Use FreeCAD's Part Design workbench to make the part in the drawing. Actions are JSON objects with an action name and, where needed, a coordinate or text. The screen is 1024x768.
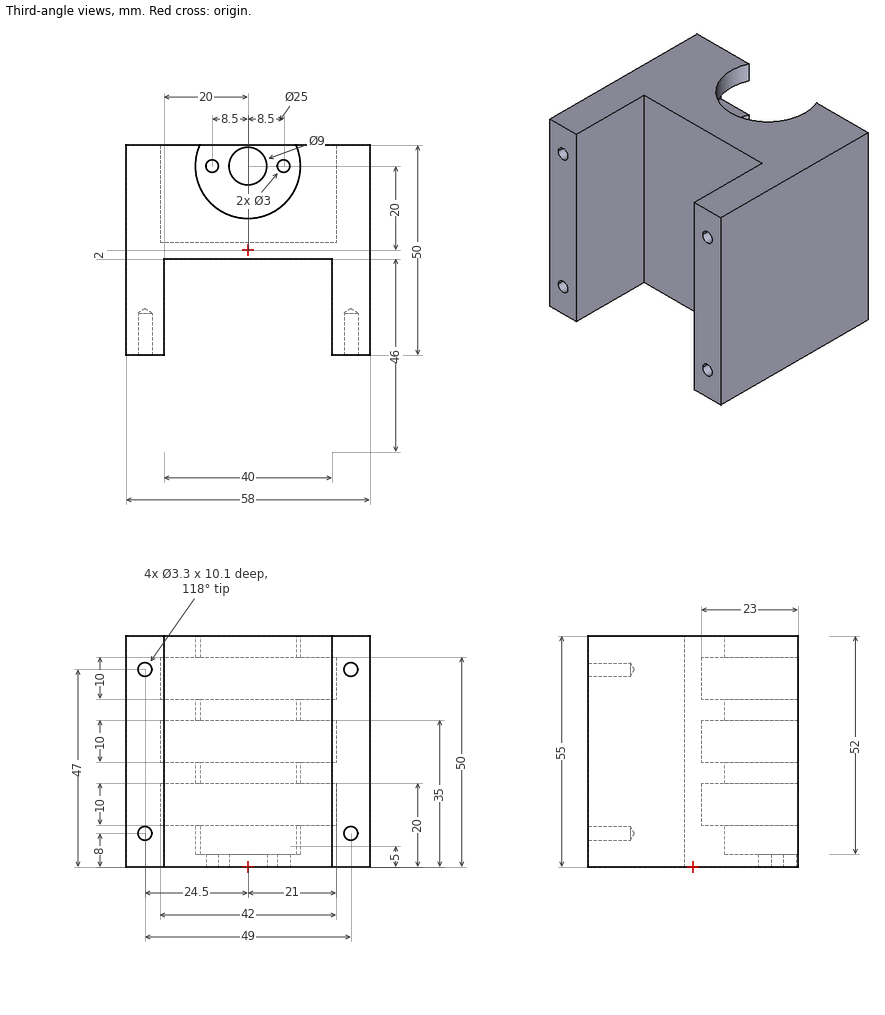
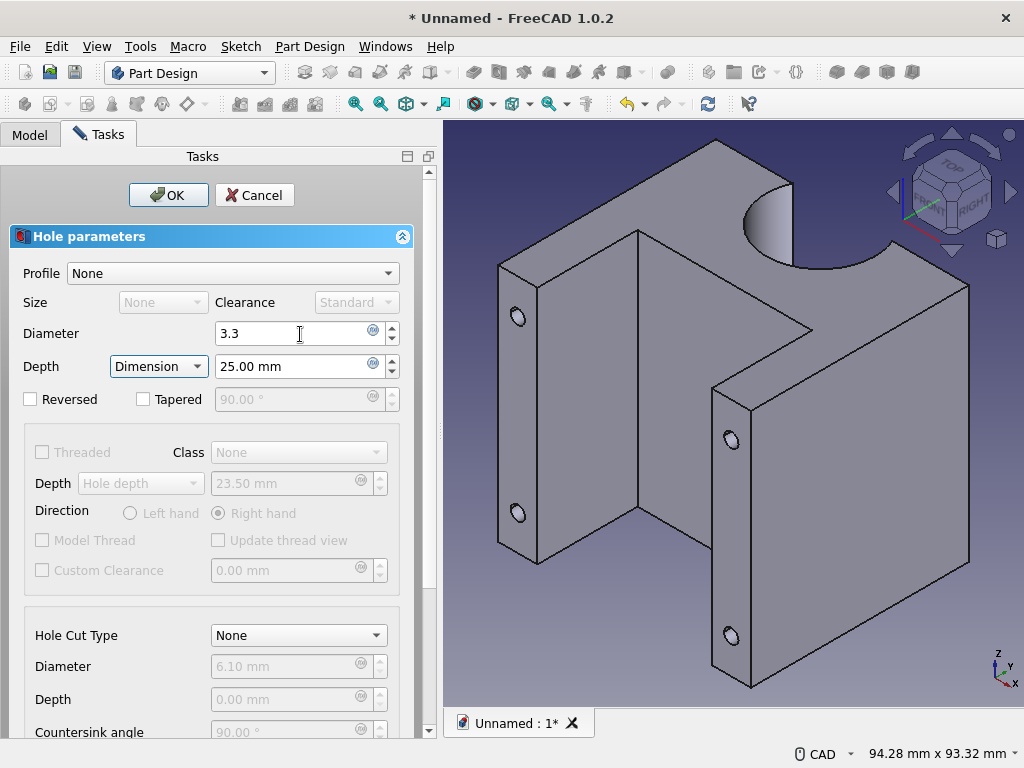
{"action": "triple_click", "coordinate": [300, 366]}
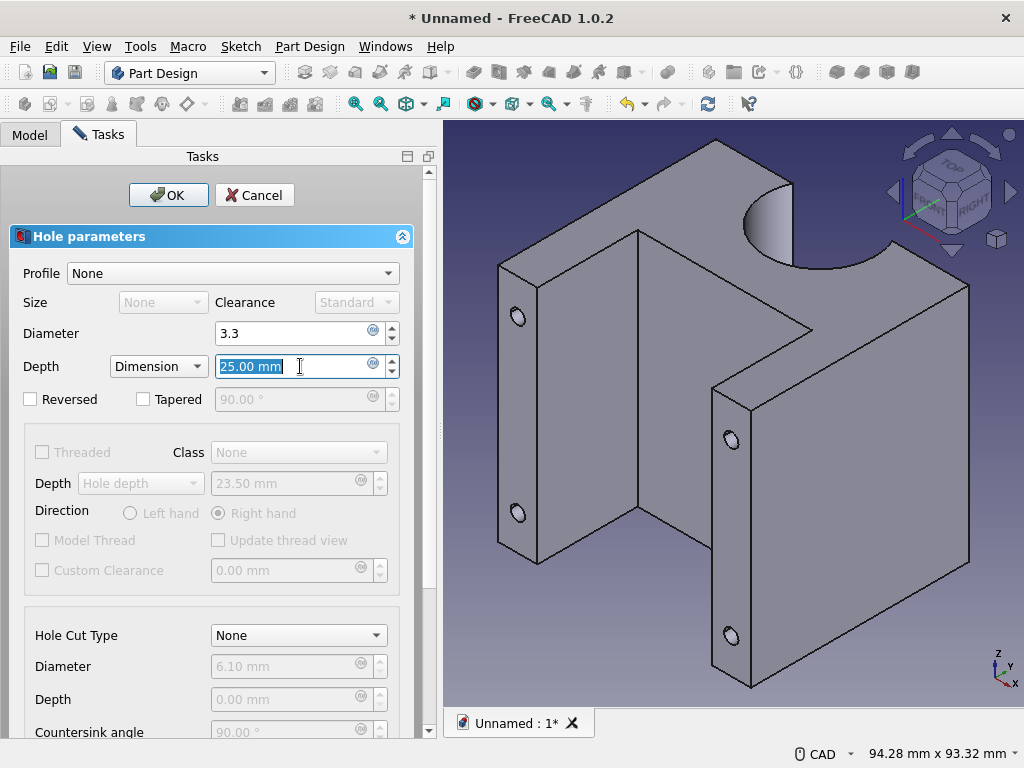
{"action": "type", "text": "10.1"}
{"action": "key", "text": "Tab"}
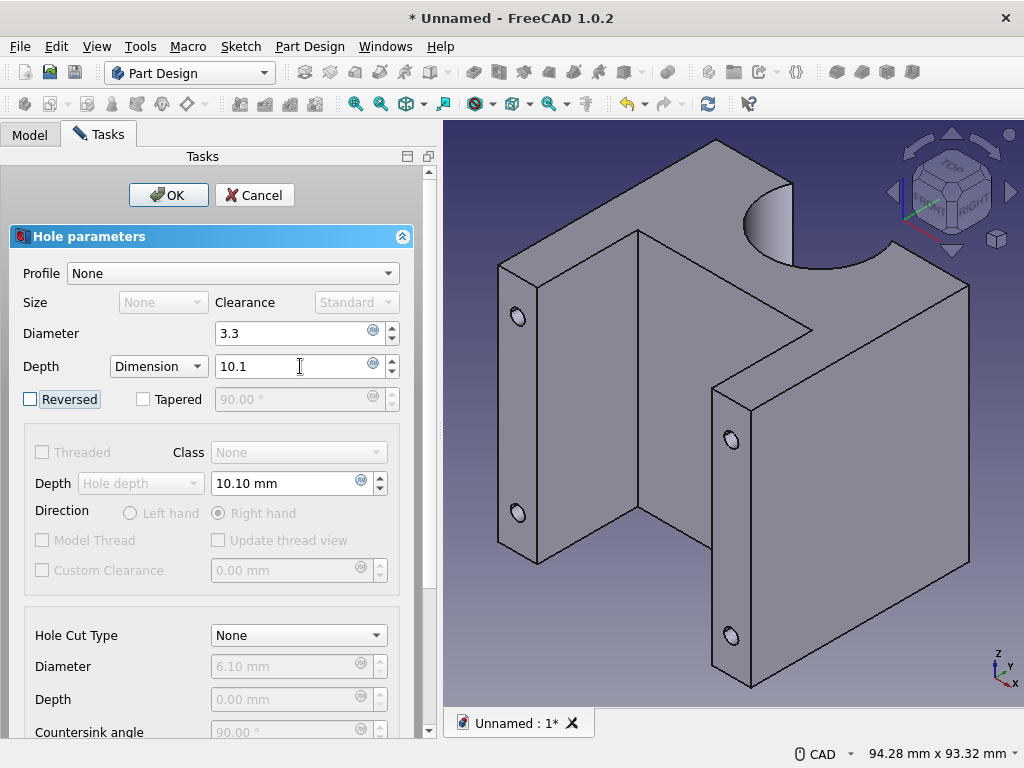
{"action": "left_click", "coordinate": [169, 195]}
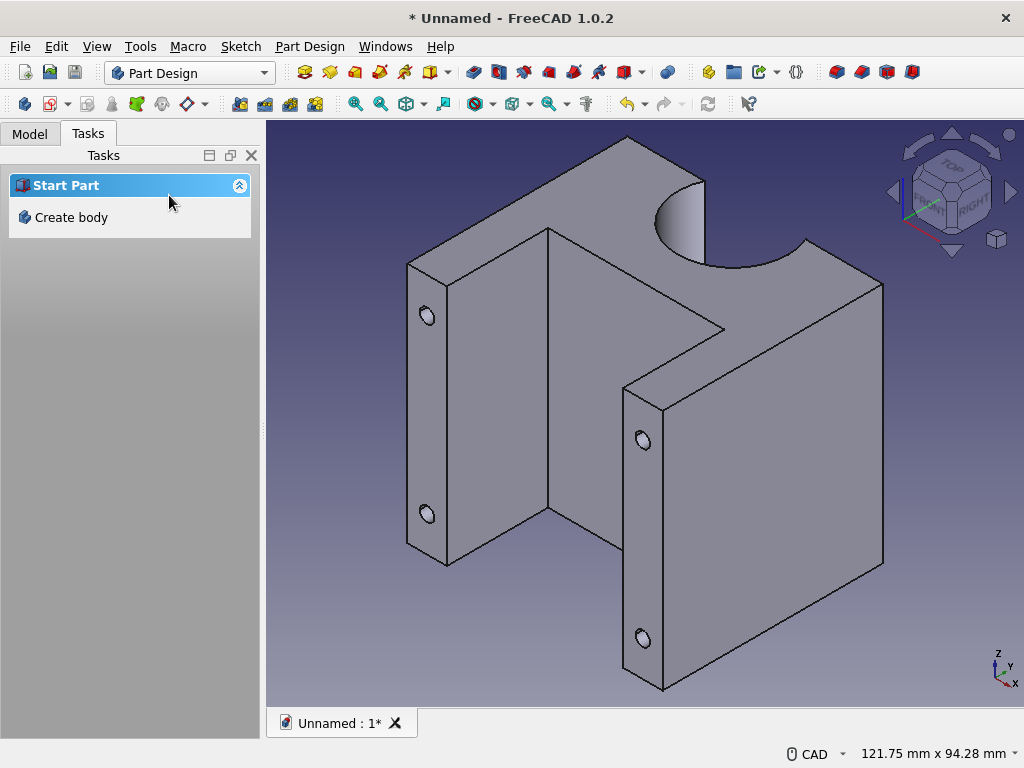
{"action": "key", "text": "4"}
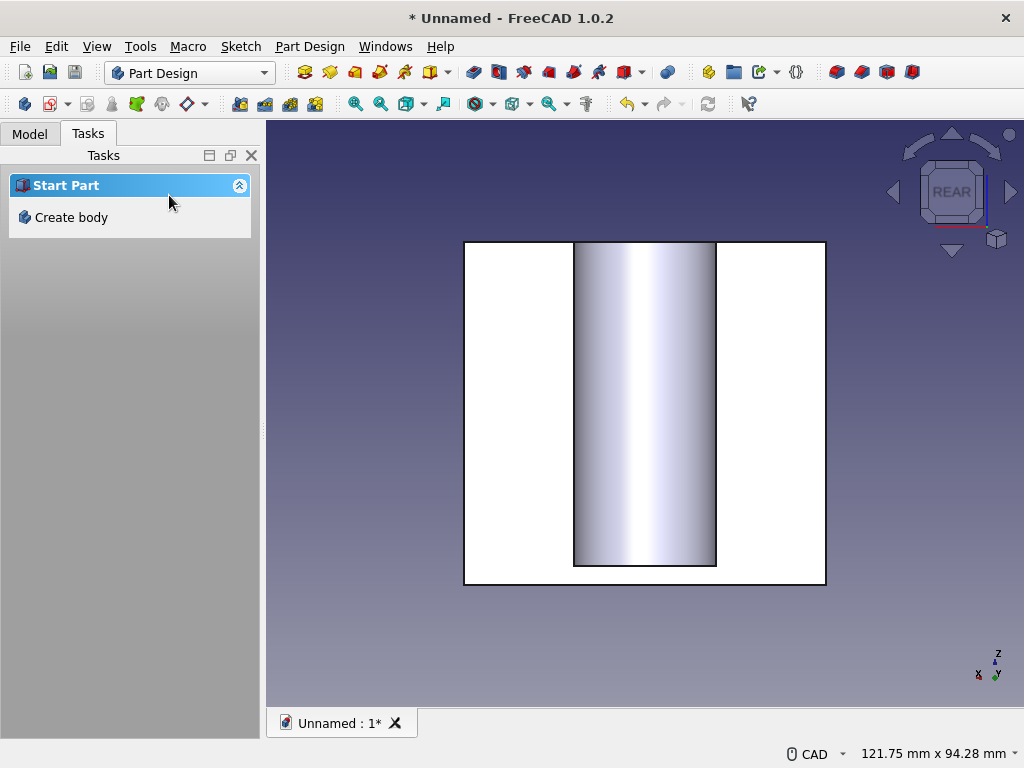
{"action": "left_click", "coordinate": [542, 315]}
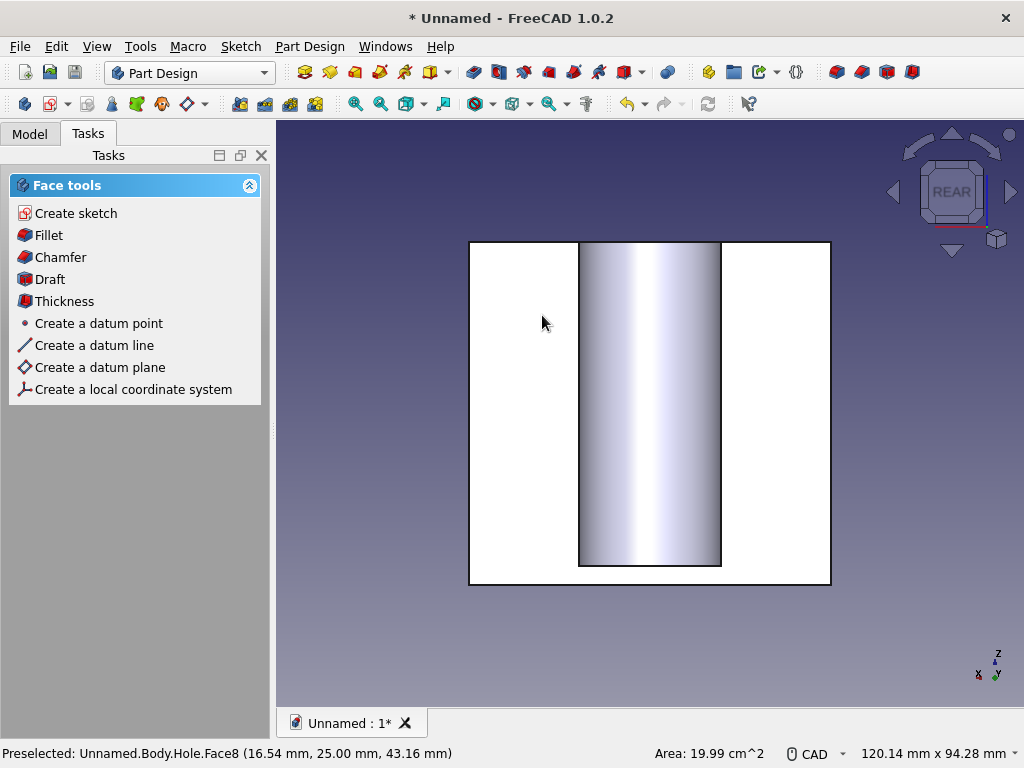
{"action": "left_click", "coordinate": [50, 104]}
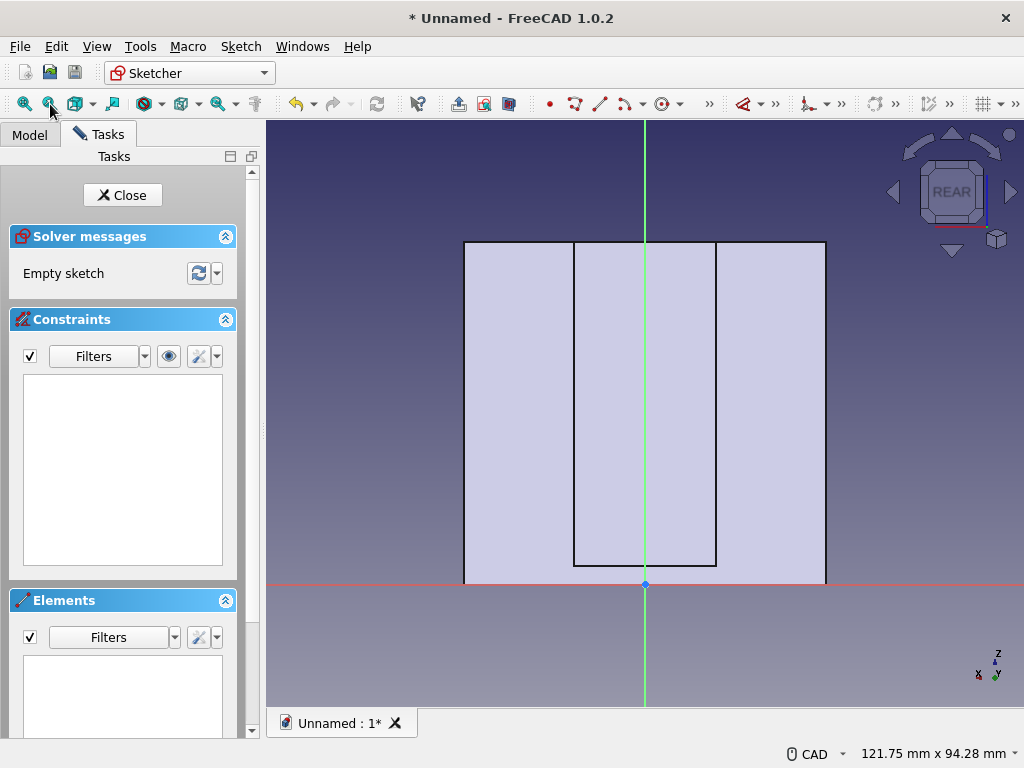
{"action": "key", "text": "g r"}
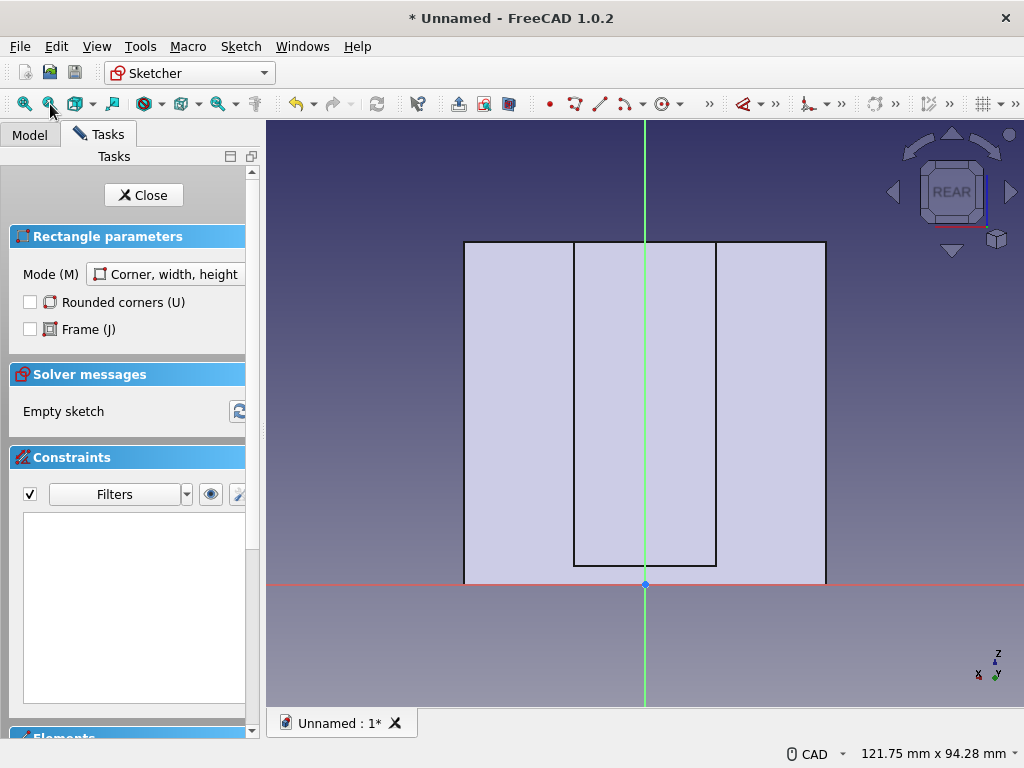
{"action": "left_click", "coordinate": [514, 460]}
{"action": "mouse_move", "coordinate": [776, 522]}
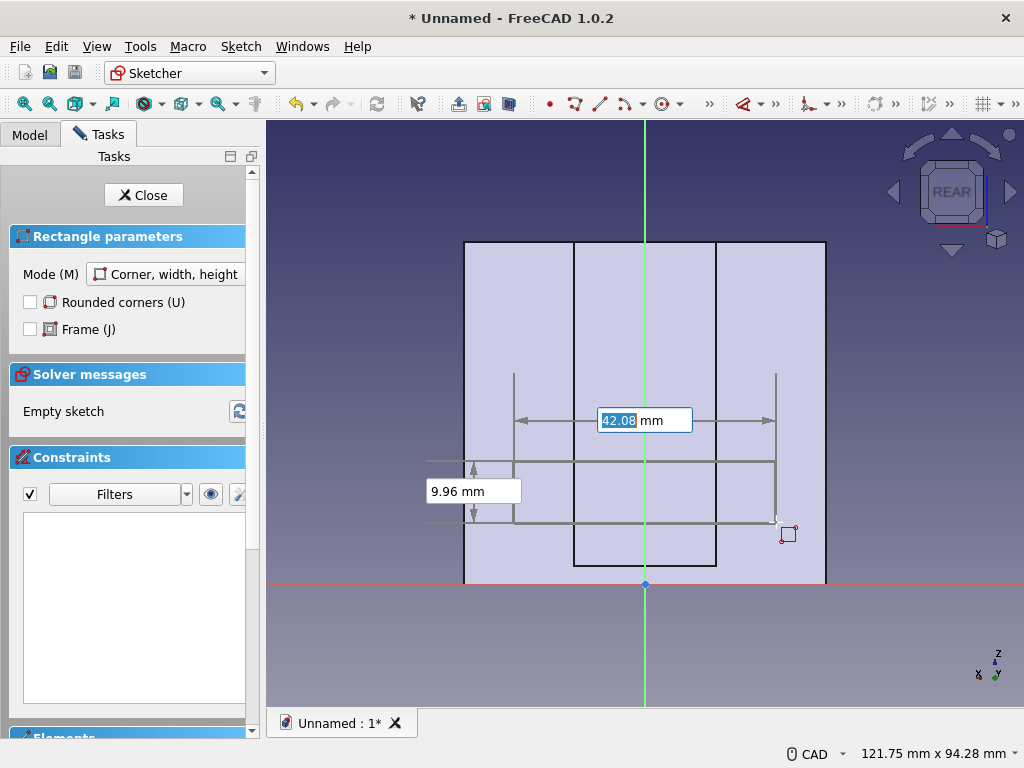
{"action": "type", "text": "42"}
{"action": "key", "text": "Tab"}
{"action": "type", "text": "10"}
{"action": "key", "text": "Return"}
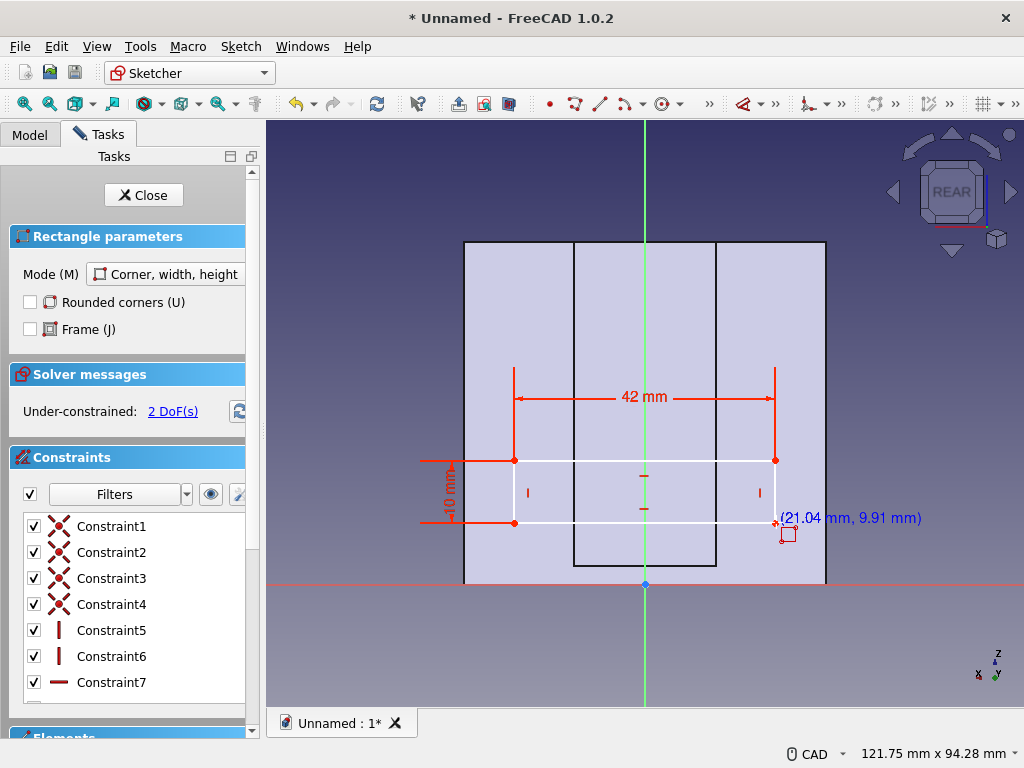
{"action": "left_click", "coordinate": [514, 367]}
{"action": "mouse_move", "coordinate": [776, 429]}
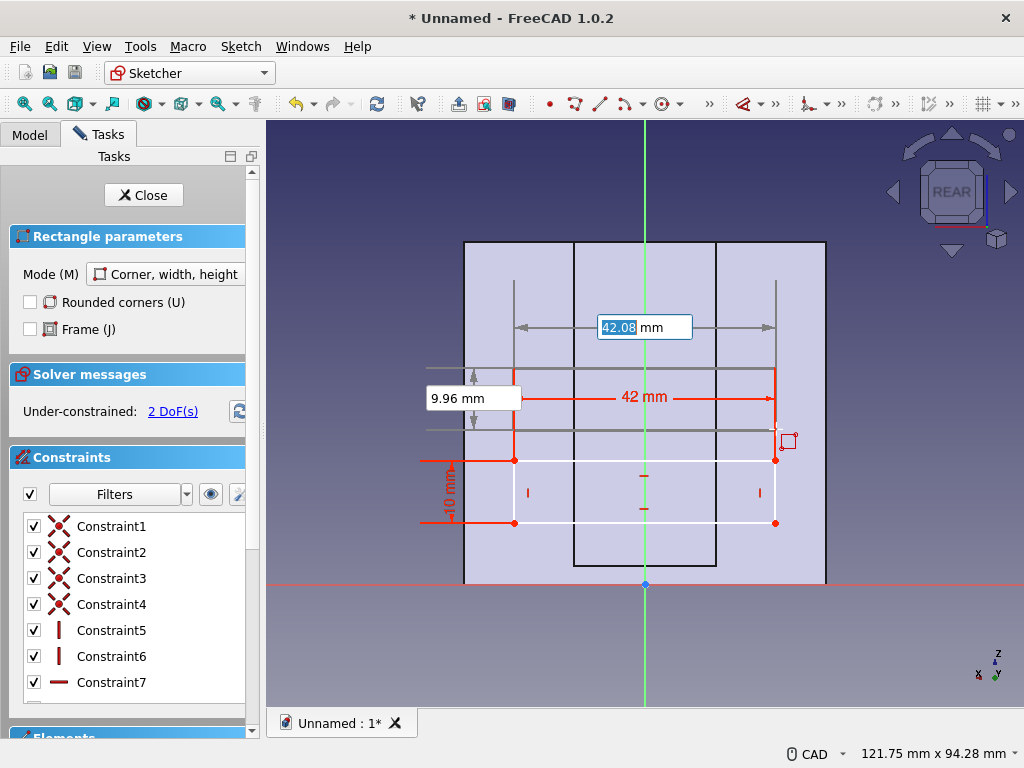
{"action": "type", "text": "42"}
{"action": "key", "text": "Tab"}
{"action": "type", "text": "10"}
{"action": "key", "text": "Return"}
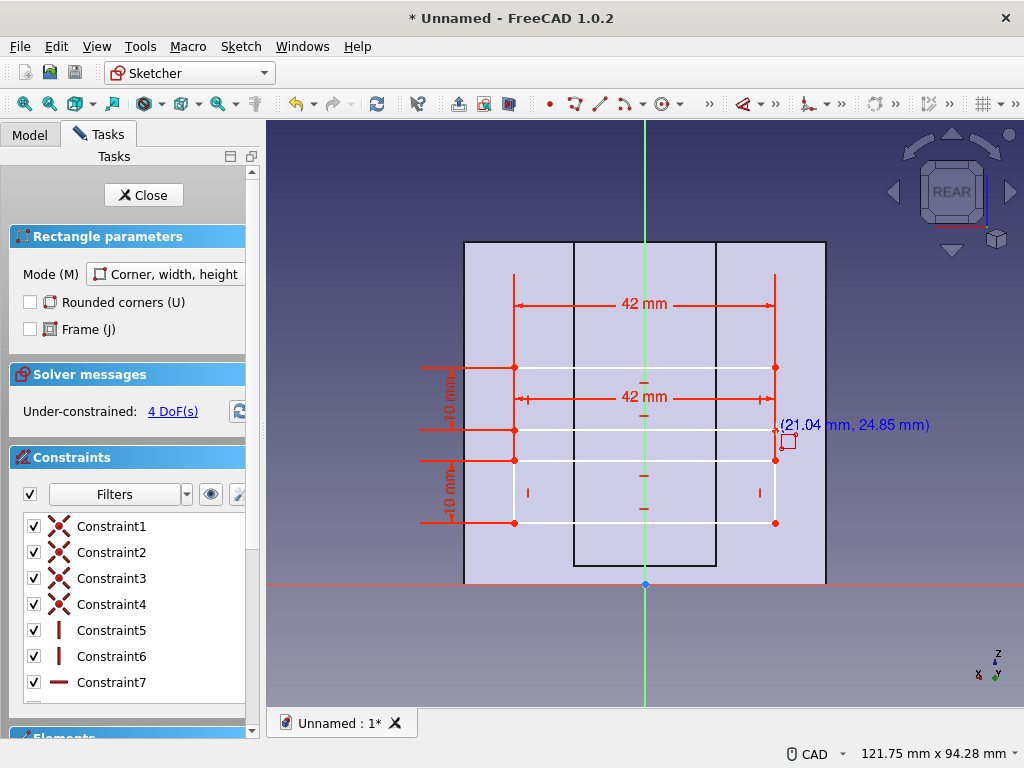
{"action": "left_click", "coordinate": [514, 273]}
{"action": "mouse_move", "coordinate": [776, 336]}